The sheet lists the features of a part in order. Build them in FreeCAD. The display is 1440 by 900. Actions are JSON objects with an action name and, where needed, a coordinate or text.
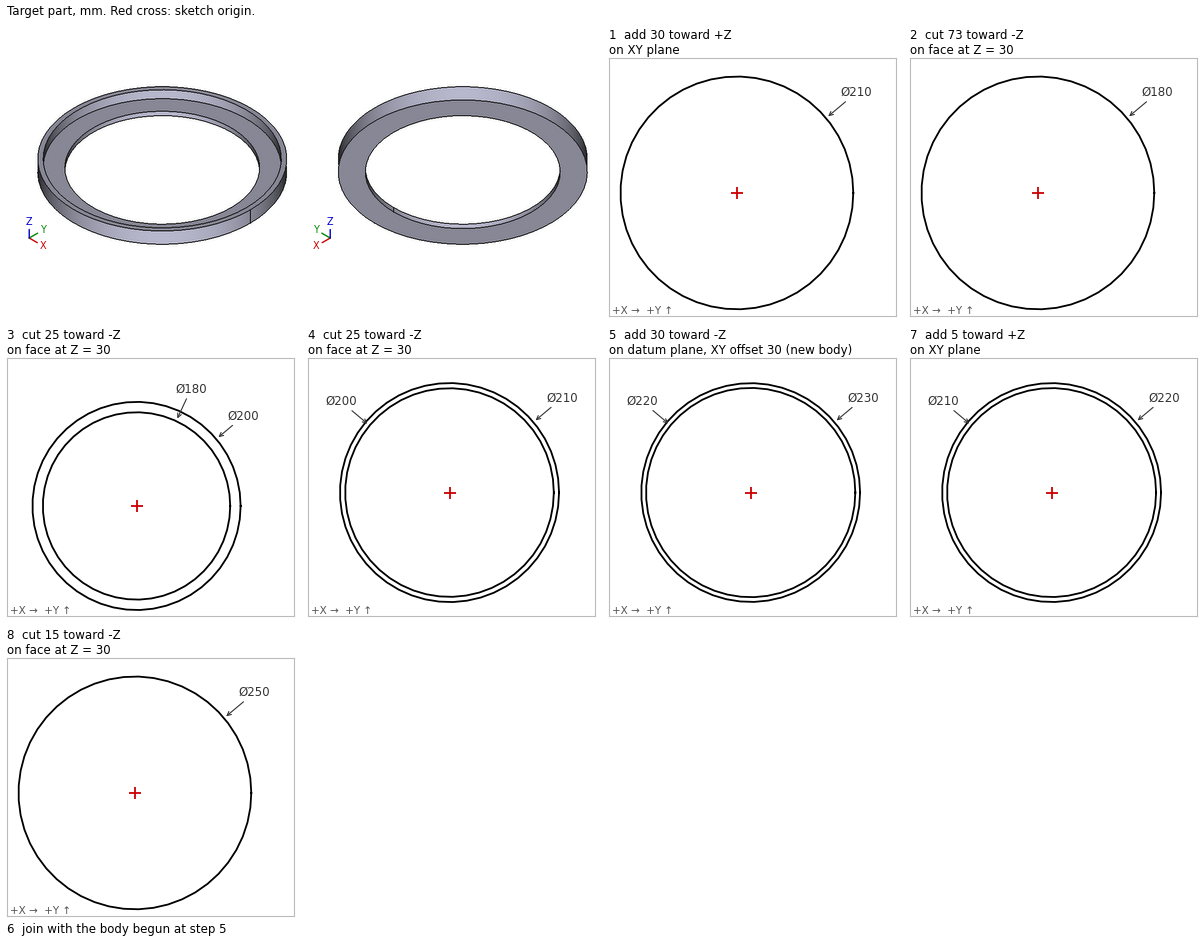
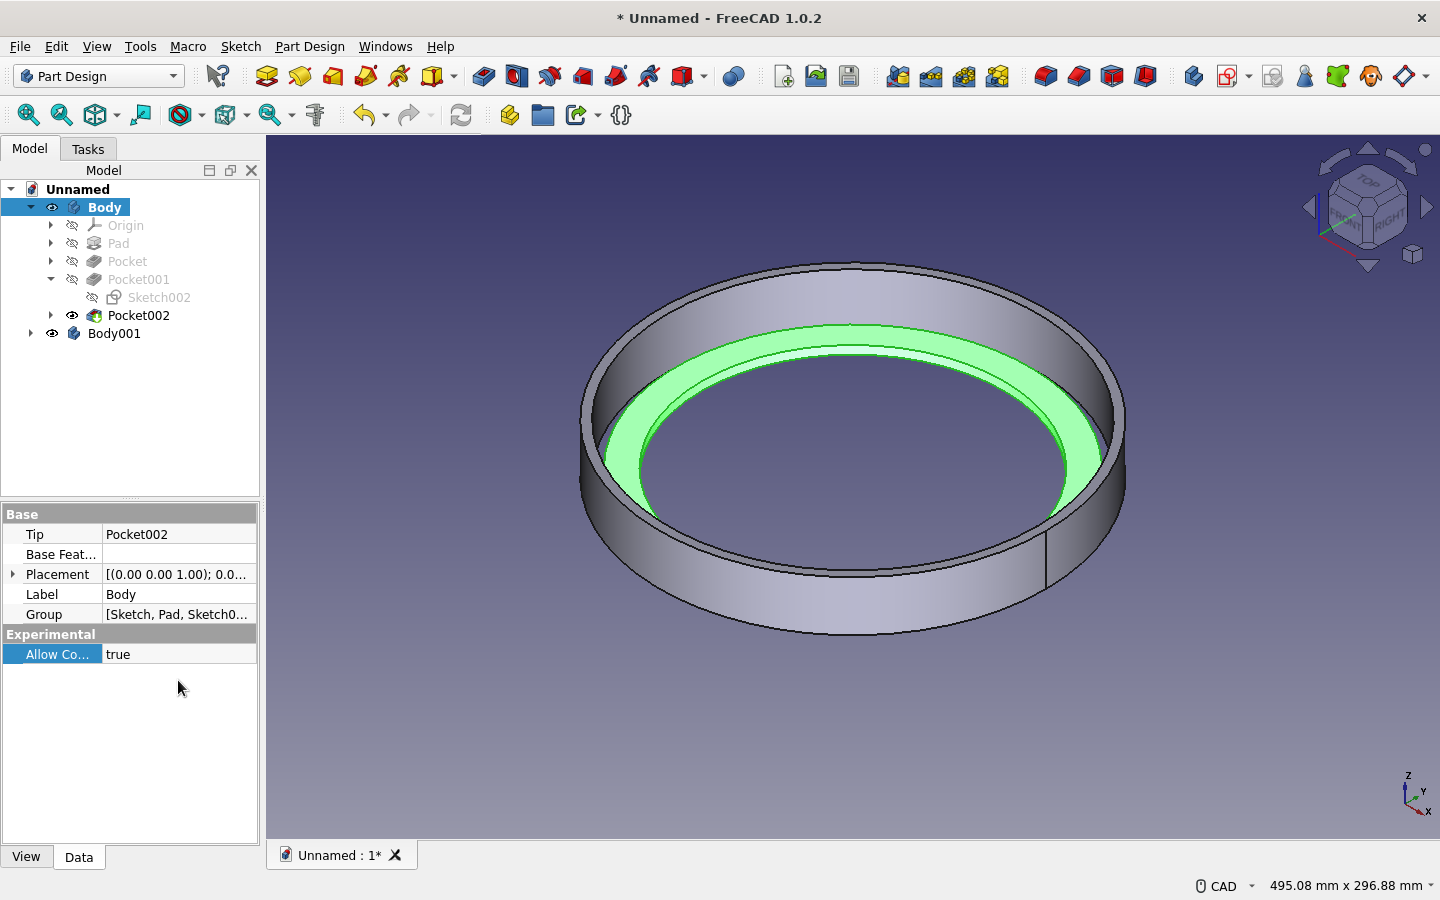
{"action": "left_click", "coordinate": [97, 333]}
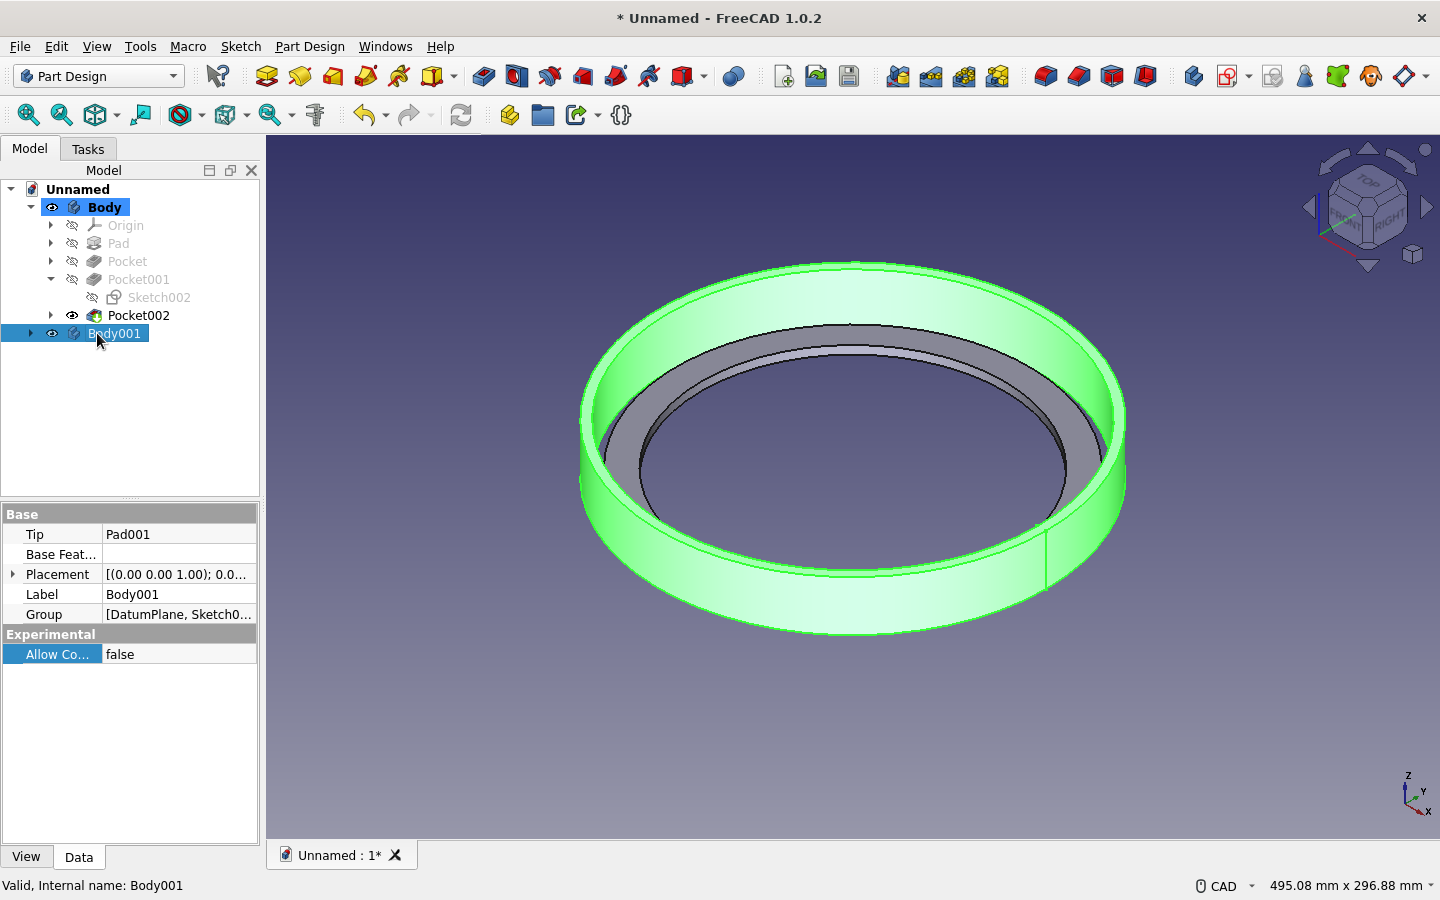
{"action": "left_click", "coordinate": [734, 76]}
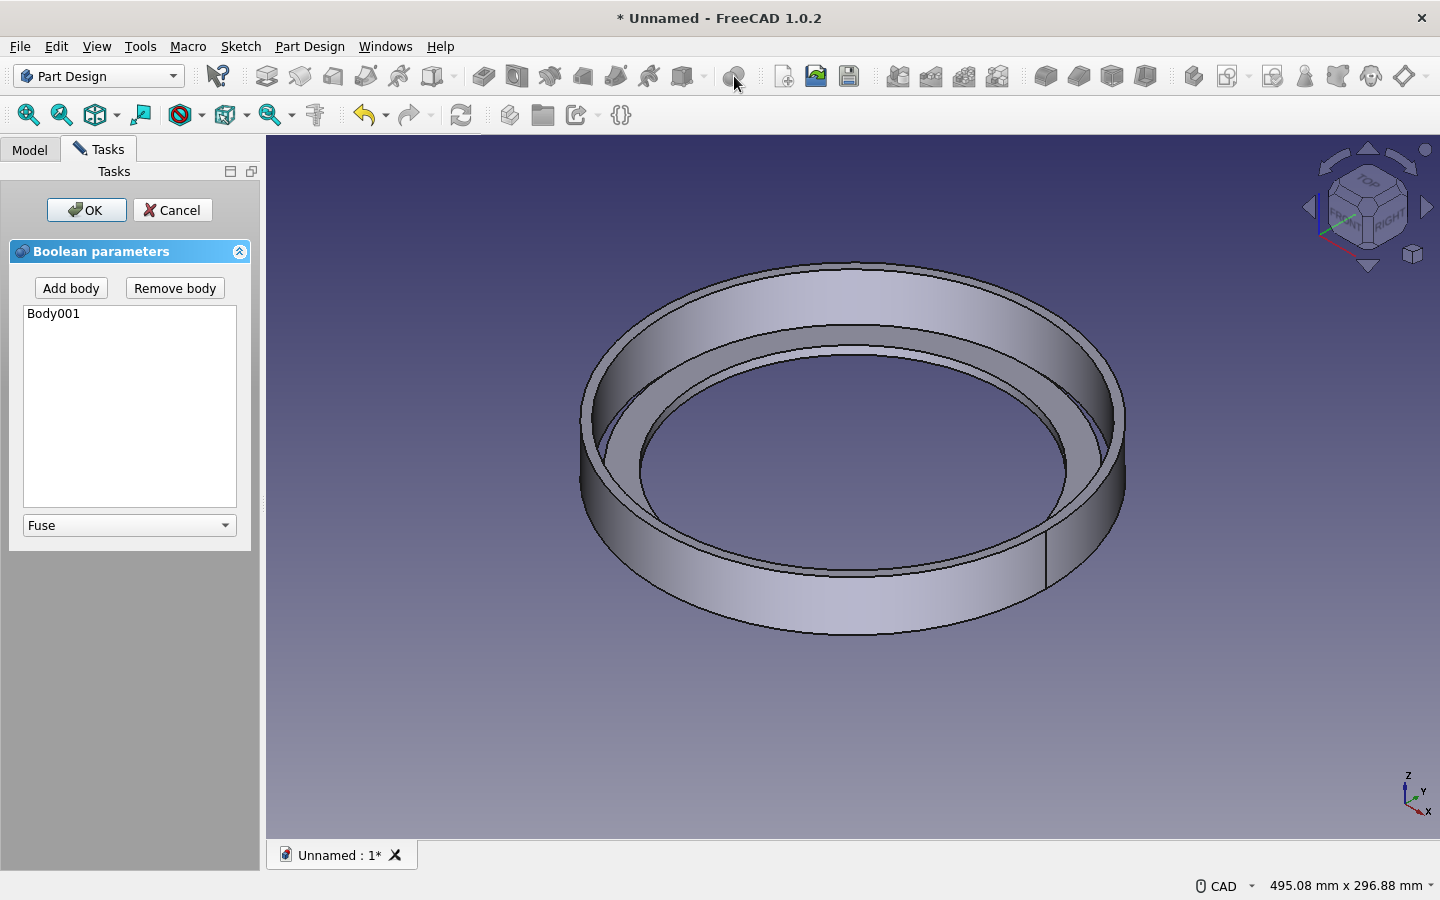
{"action": "left_click", "coordinate": [87, 210]}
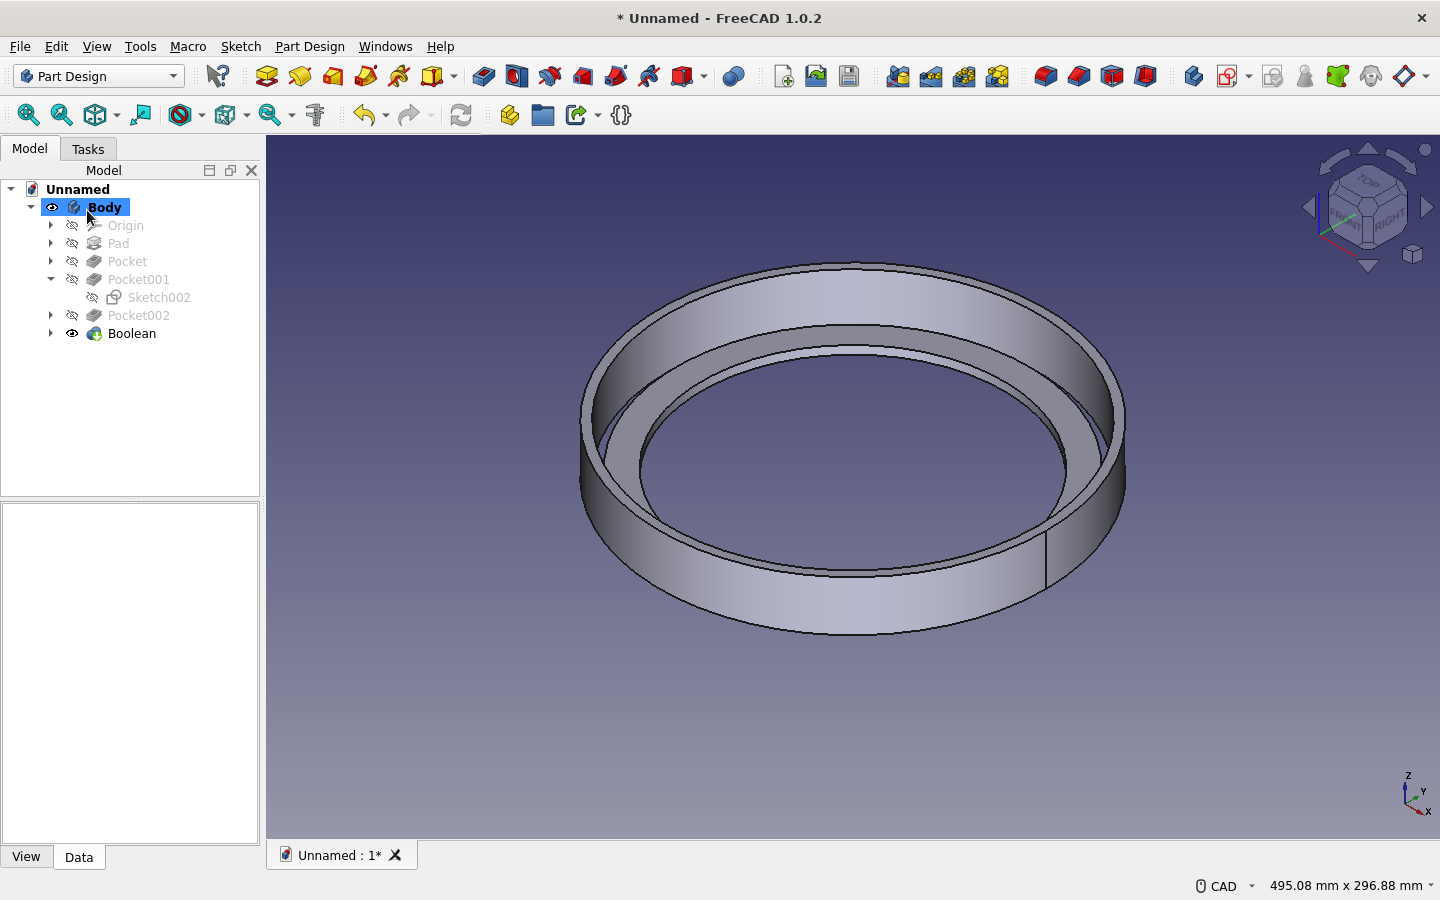
{"action": "left_click", "coordinate": [1226, 76]}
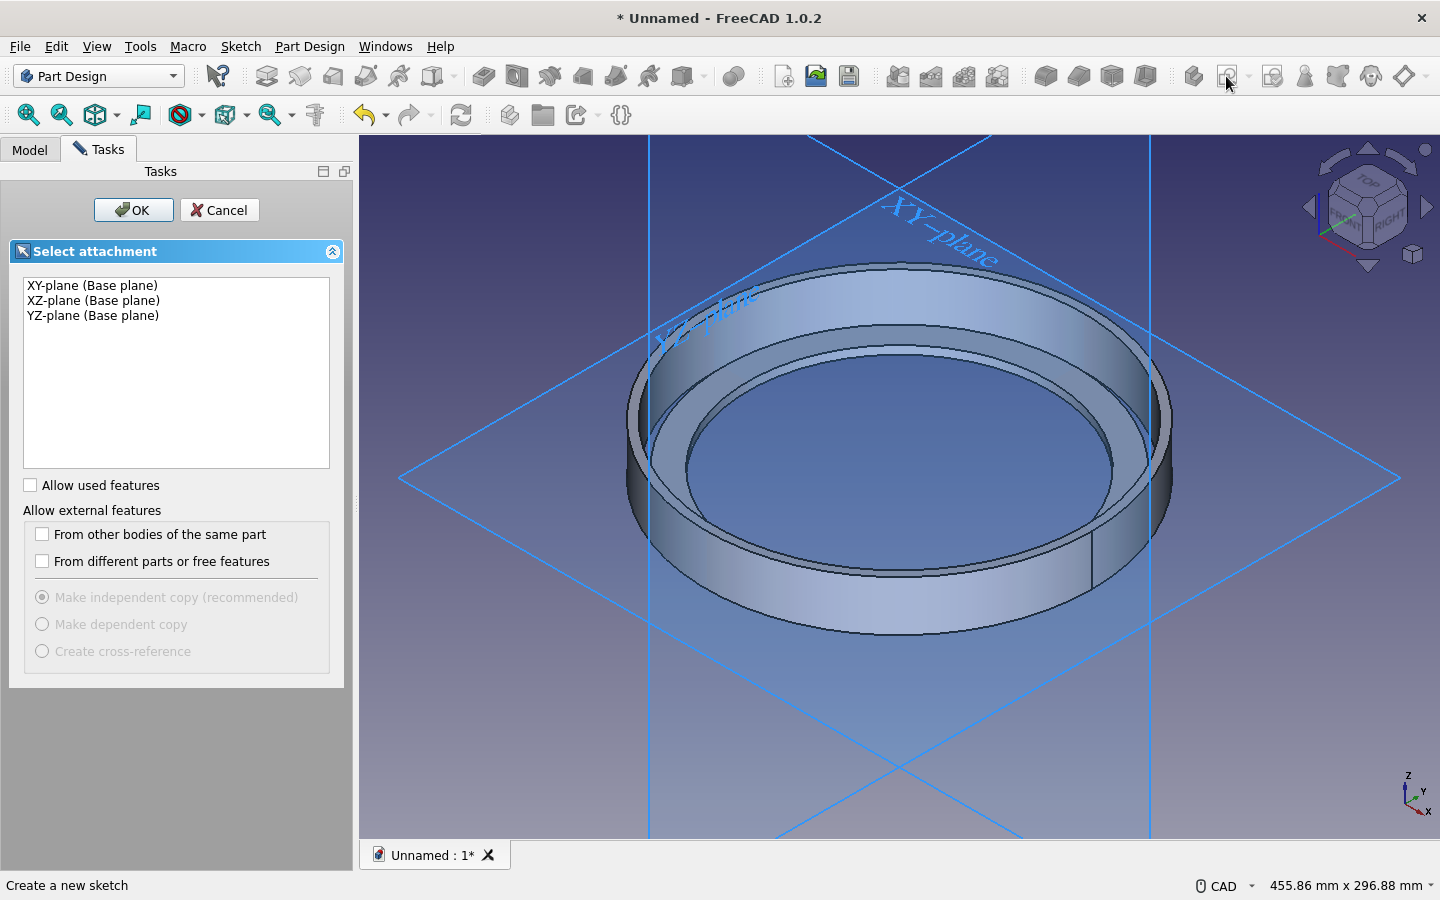
{"action": "left_click", "coordinate": [84, 286]}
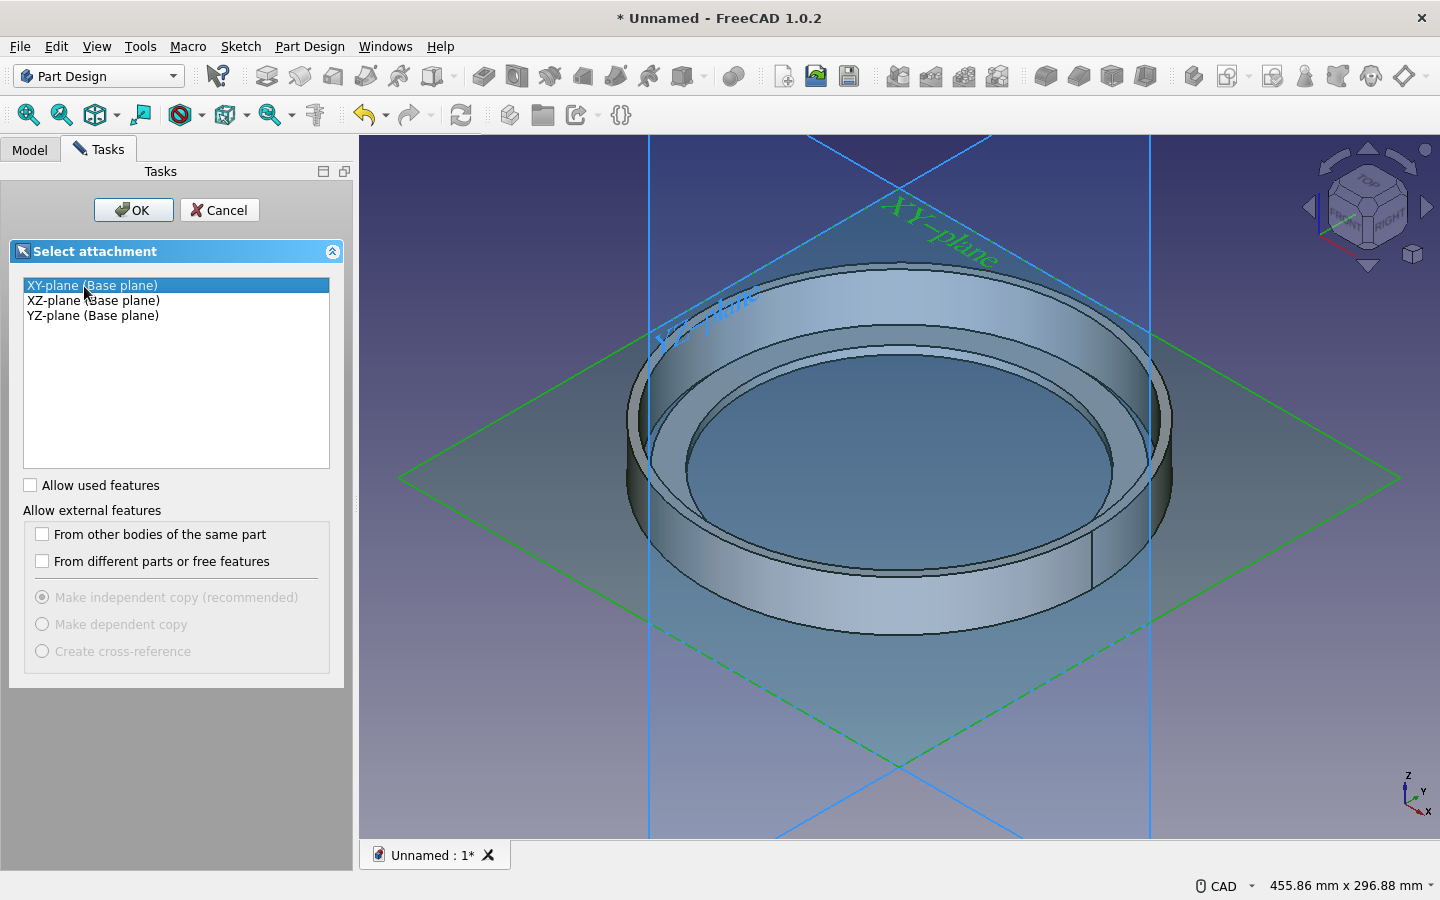
{"action": "left_click", "coordinate": [134, 210]}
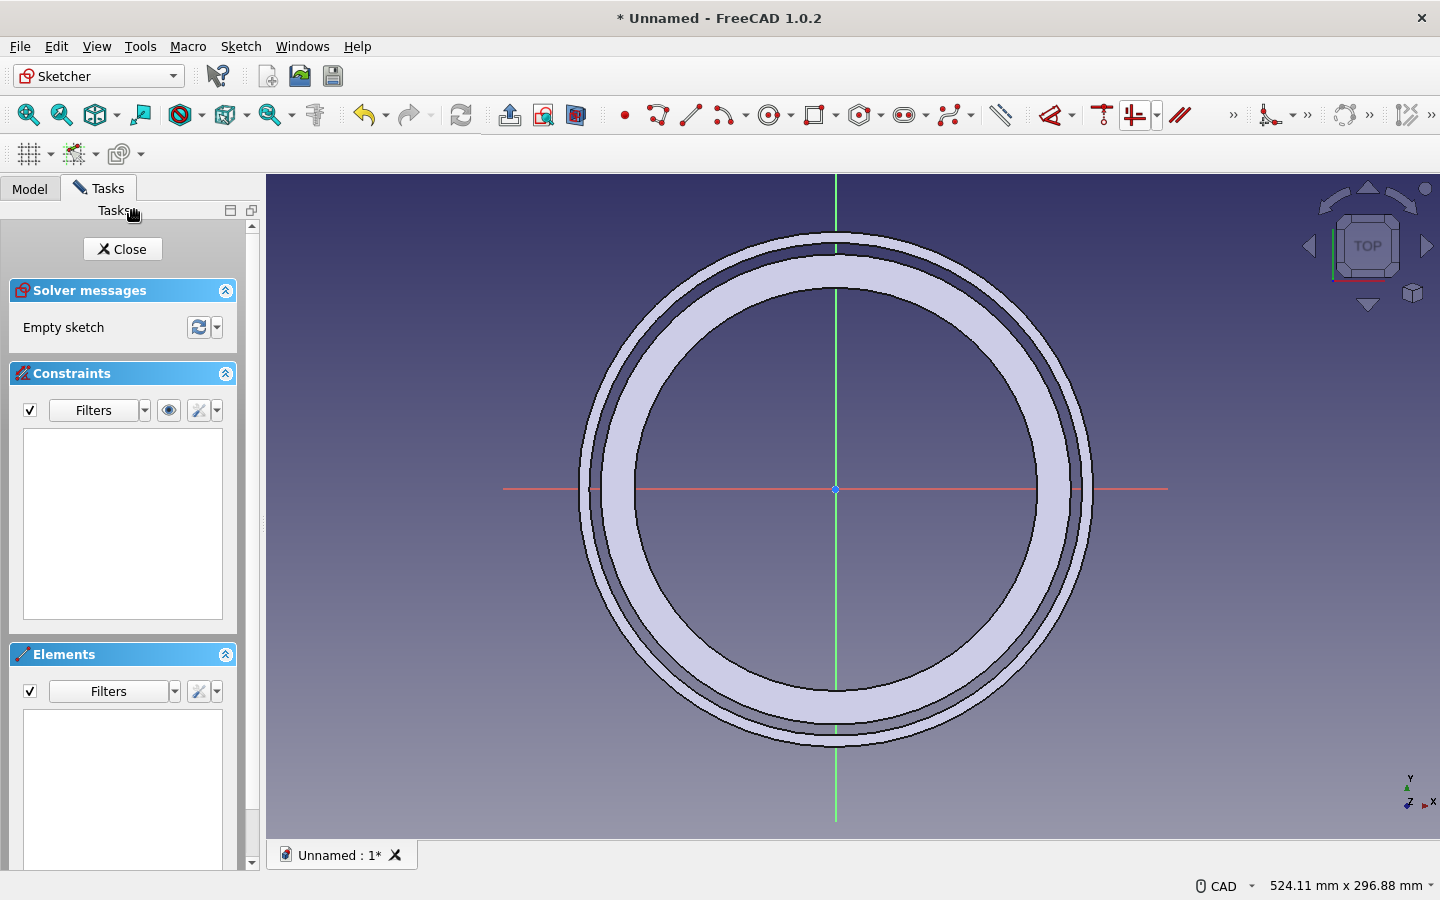
{"action": "left_click", "coordinate": [576, 116]}